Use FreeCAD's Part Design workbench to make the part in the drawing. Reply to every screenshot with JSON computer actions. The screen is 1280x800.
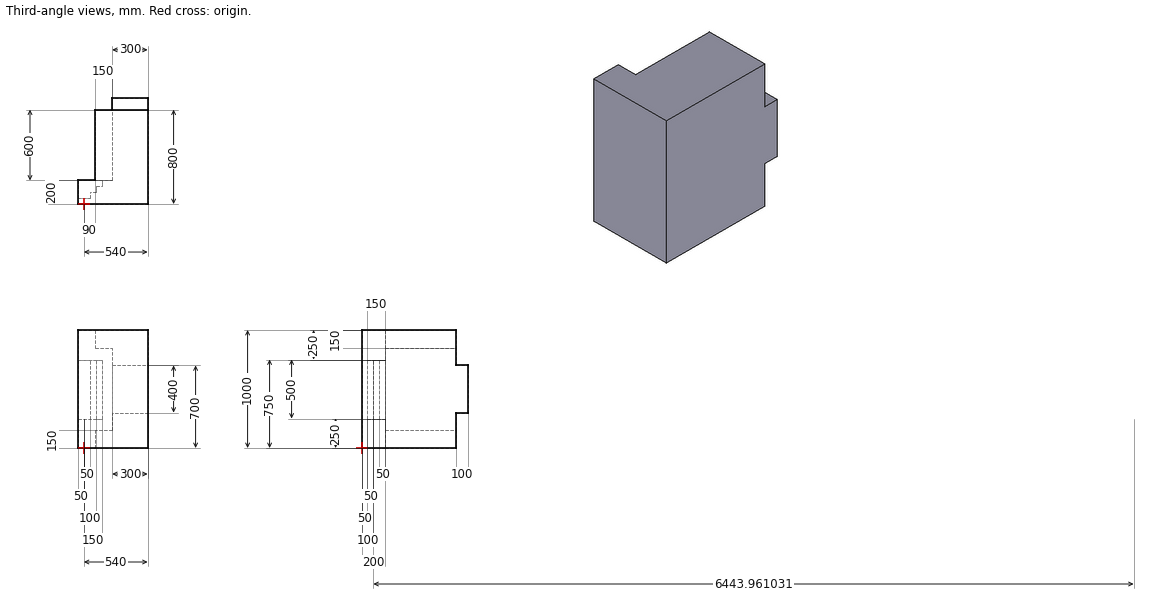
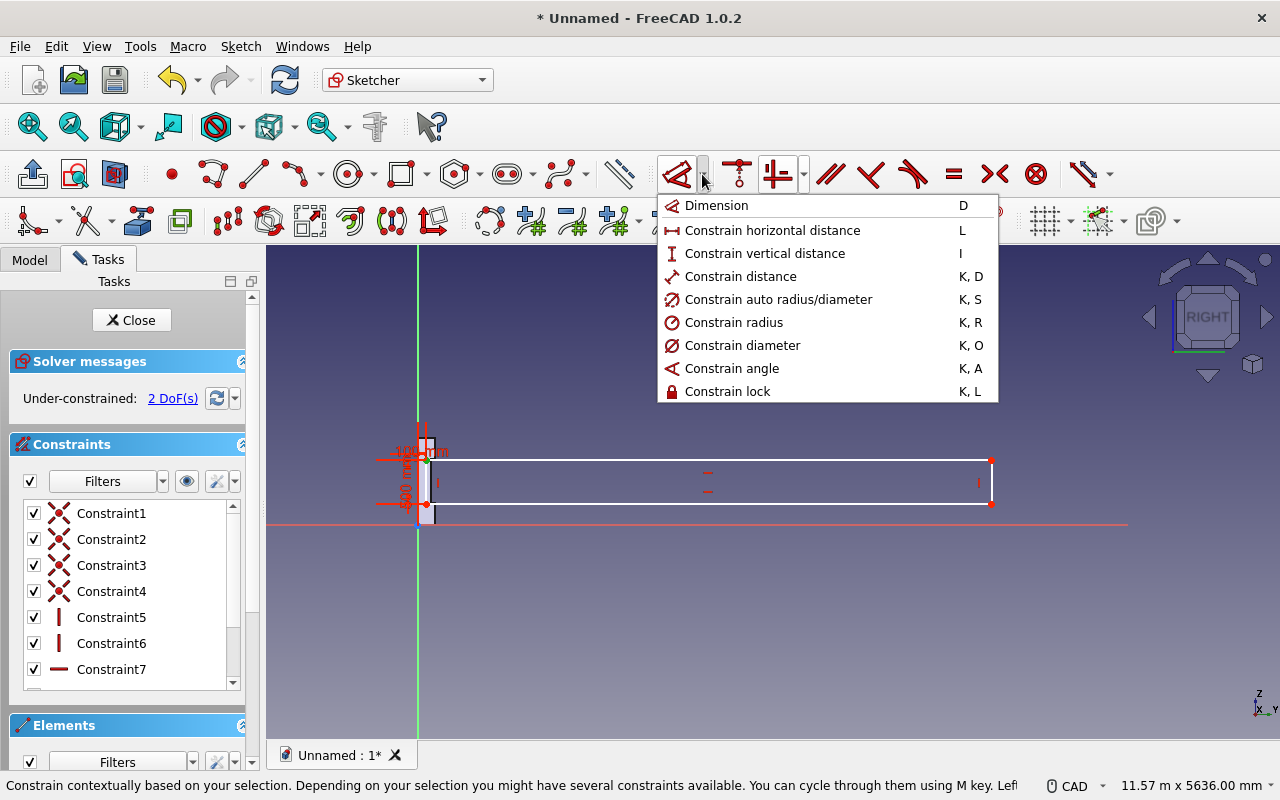
{"action": "left_click", "coordinate": [828, 254]}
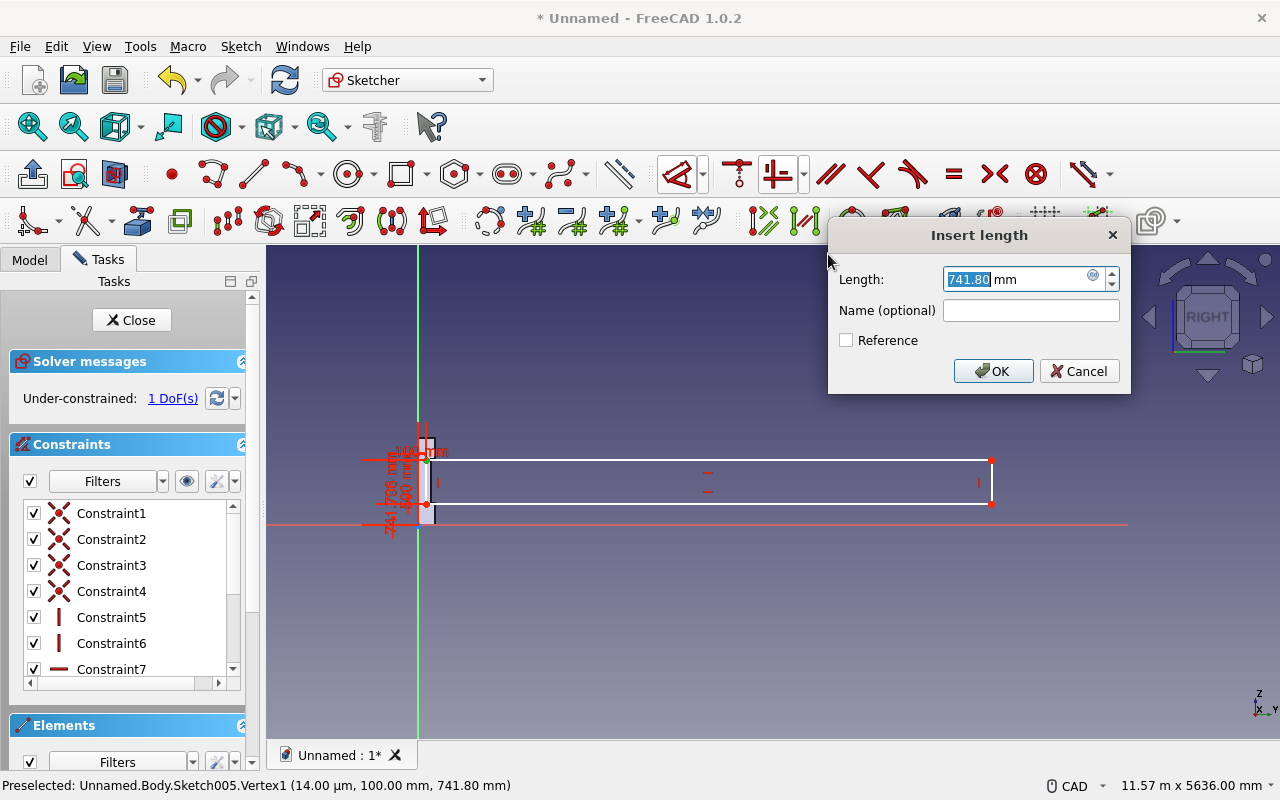
{"action": "type", "text": "750"}
{"action": "key", "text": "Return"}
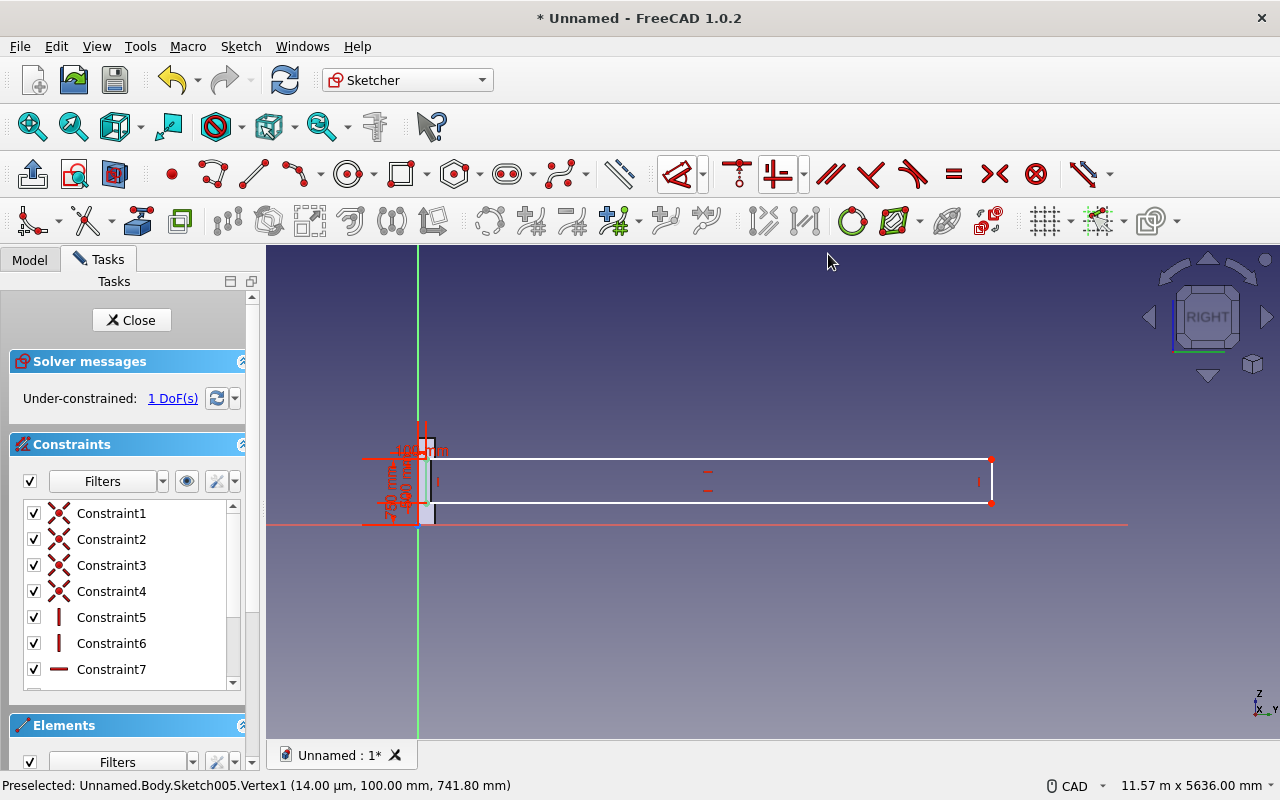
{"action": "left_click", "coordinate": [596, 503]}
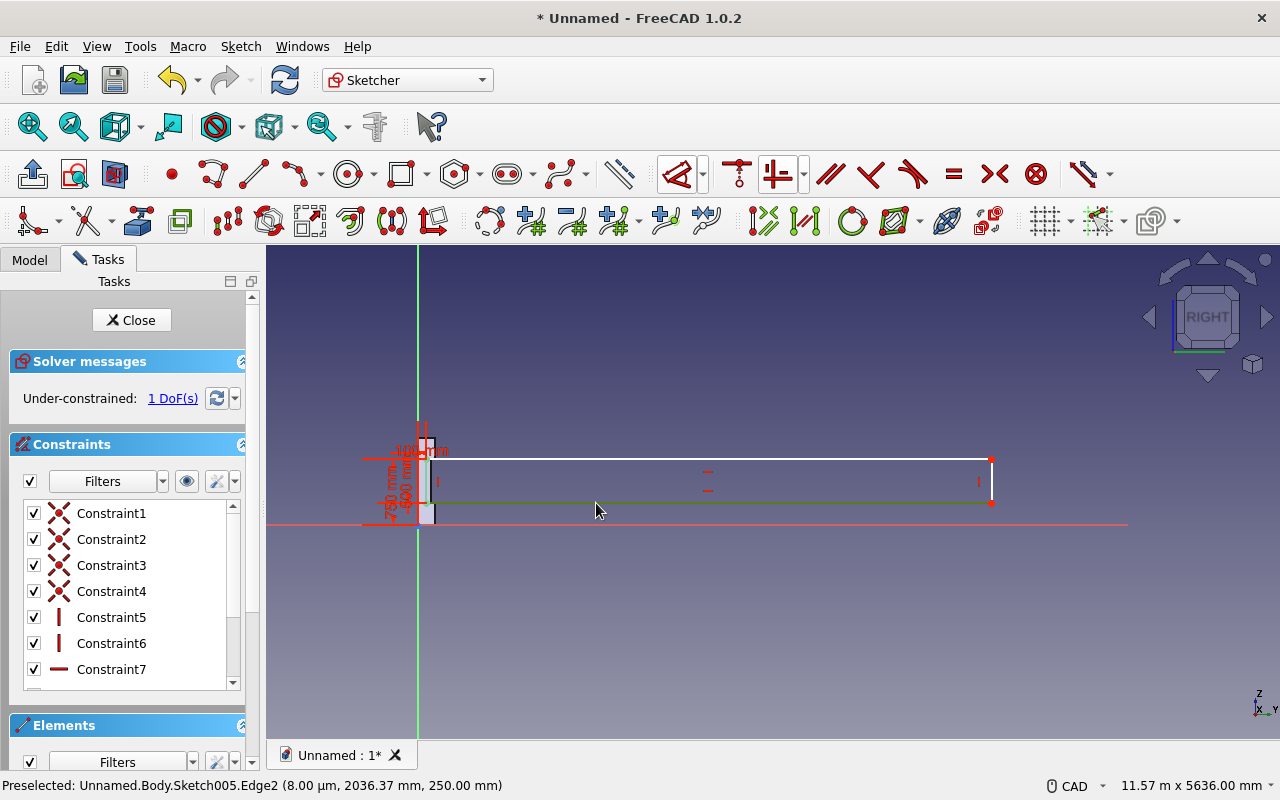
{"action": "key", "text": "l"}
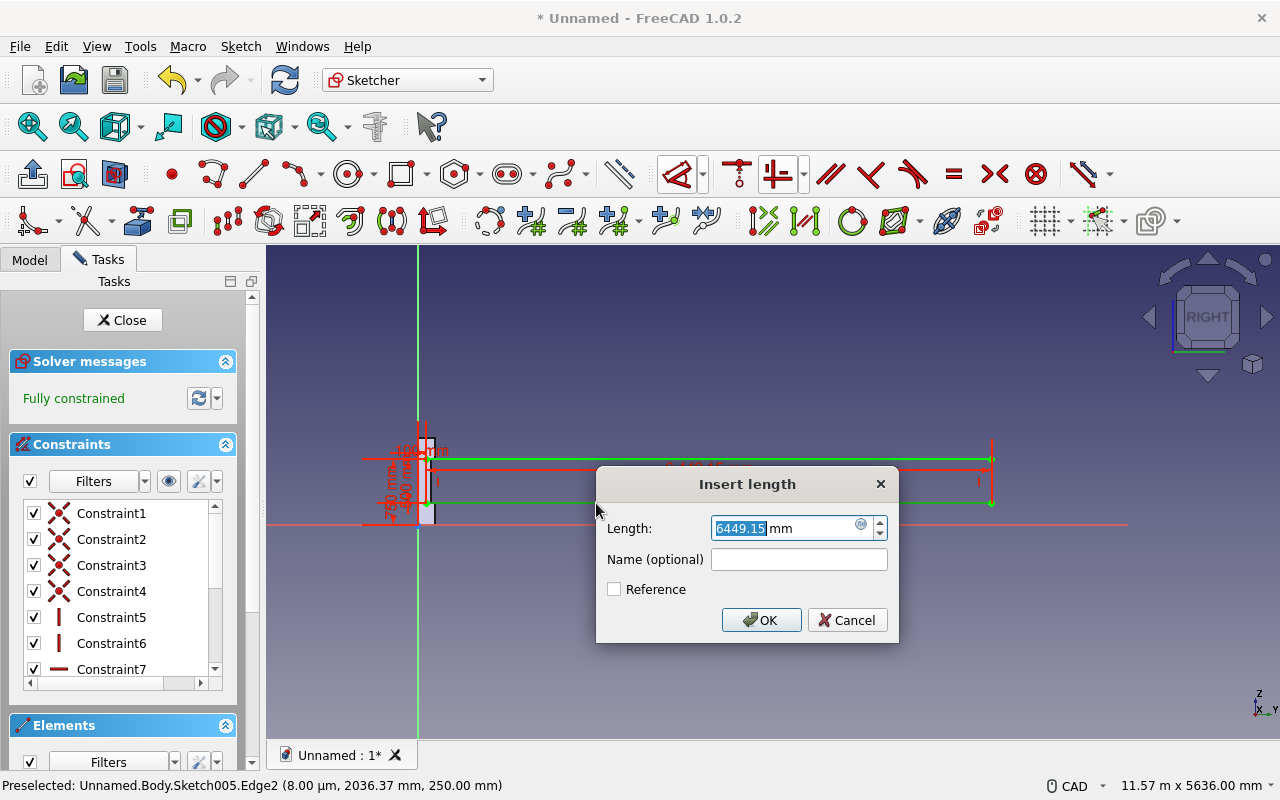
{"action": "type", "text": "6443.961031"}
{"action": "key", "text": "Return"}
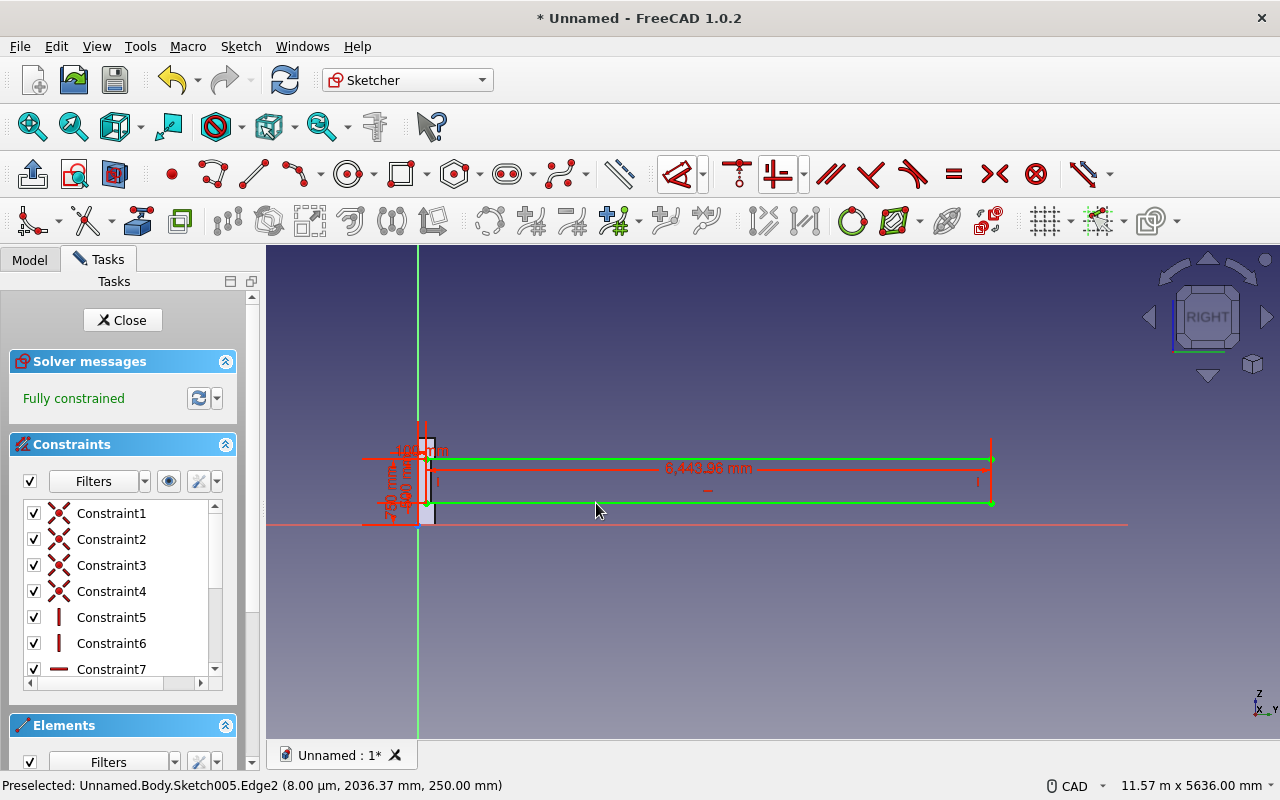
{"action": "left_click", "coordinate": [123, 320]}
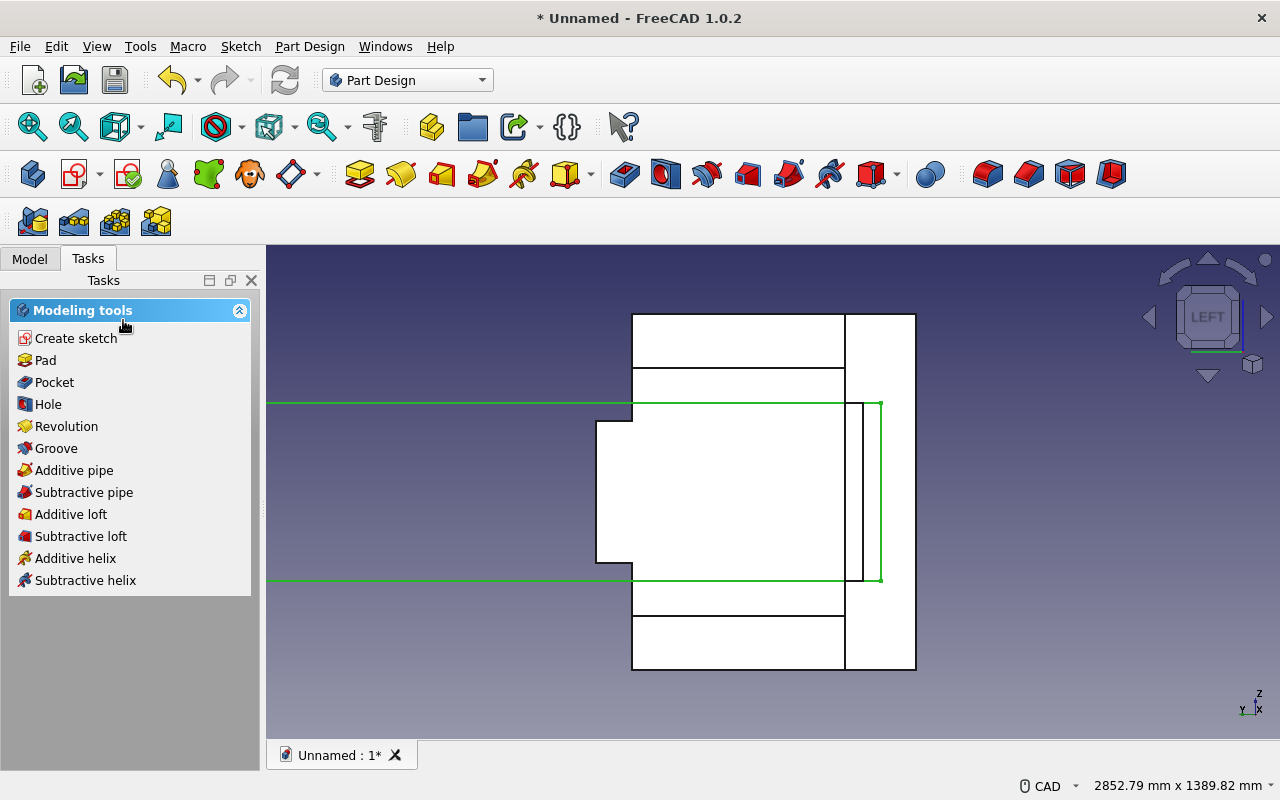
{"action": "left_click", "coordinate": [625, 174]}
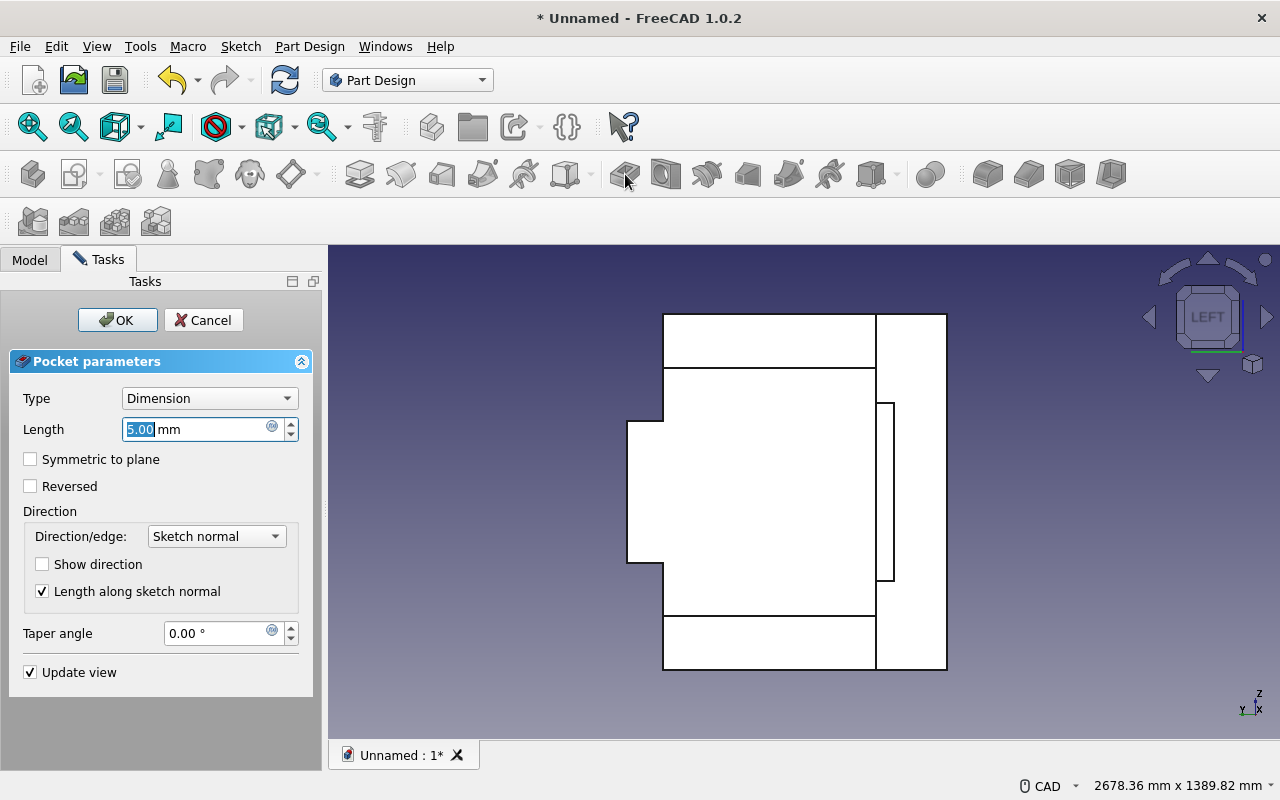
{"action": "left_click", "coordinate": [210, 398]}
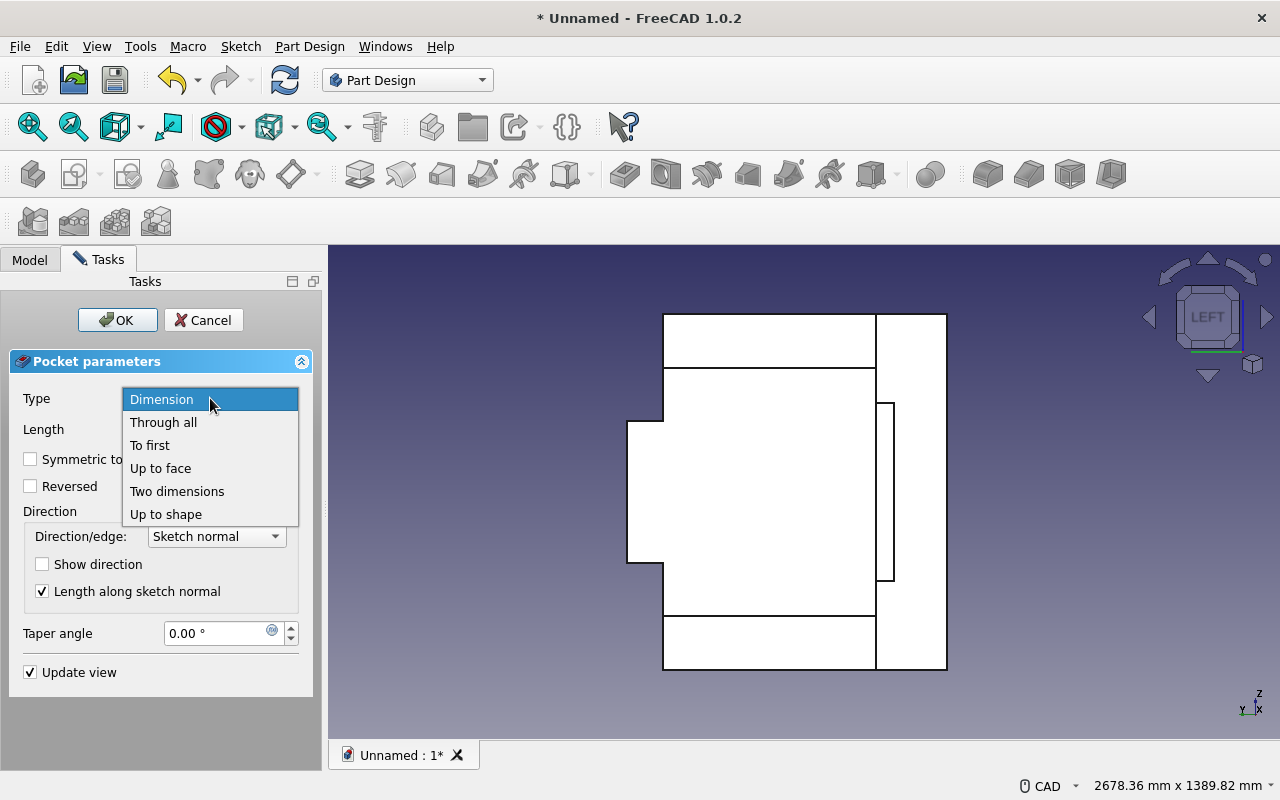
{"action": "left_click", "coordinate": [208, 492]}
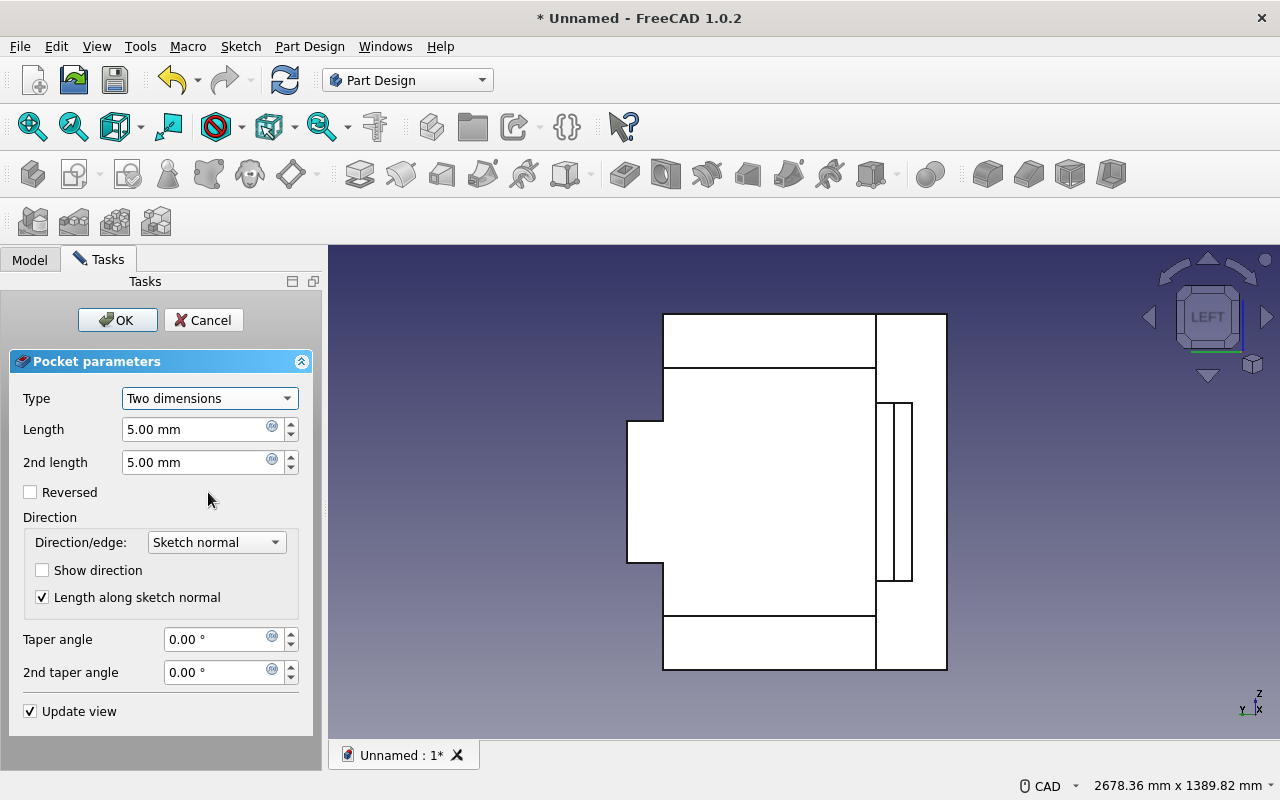
{"action": "triple_click", "coordinate": [204, 430]}